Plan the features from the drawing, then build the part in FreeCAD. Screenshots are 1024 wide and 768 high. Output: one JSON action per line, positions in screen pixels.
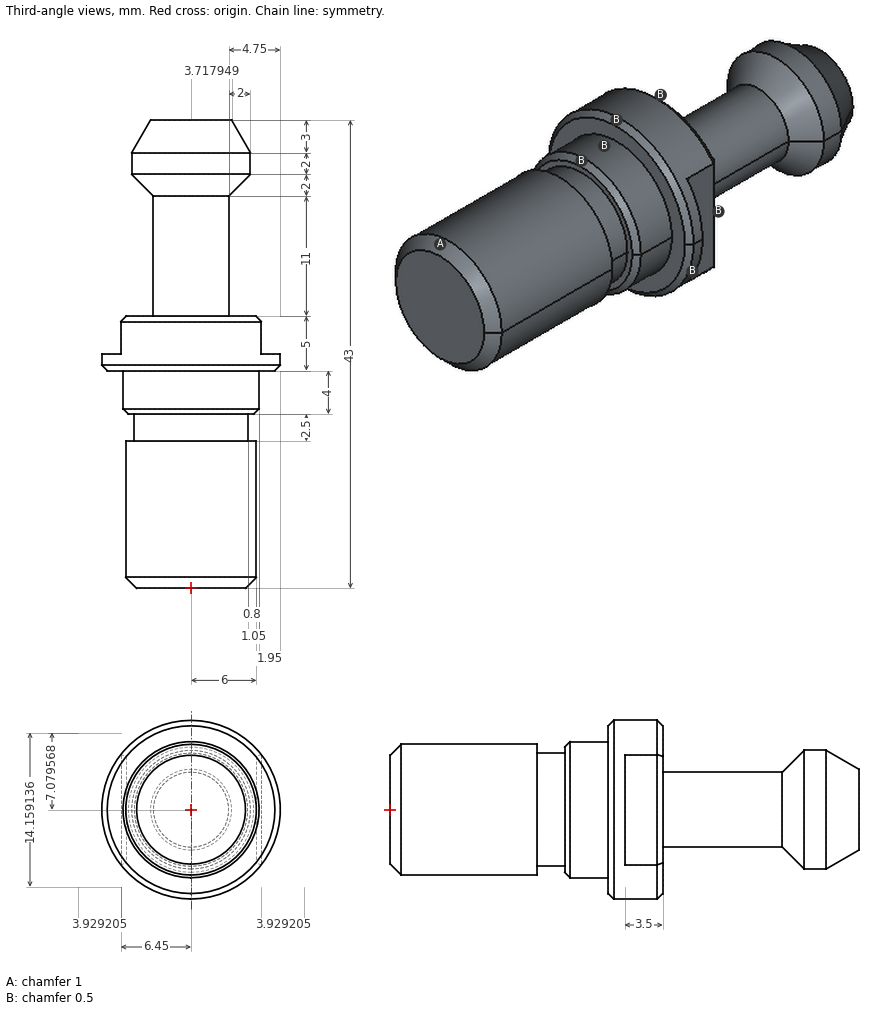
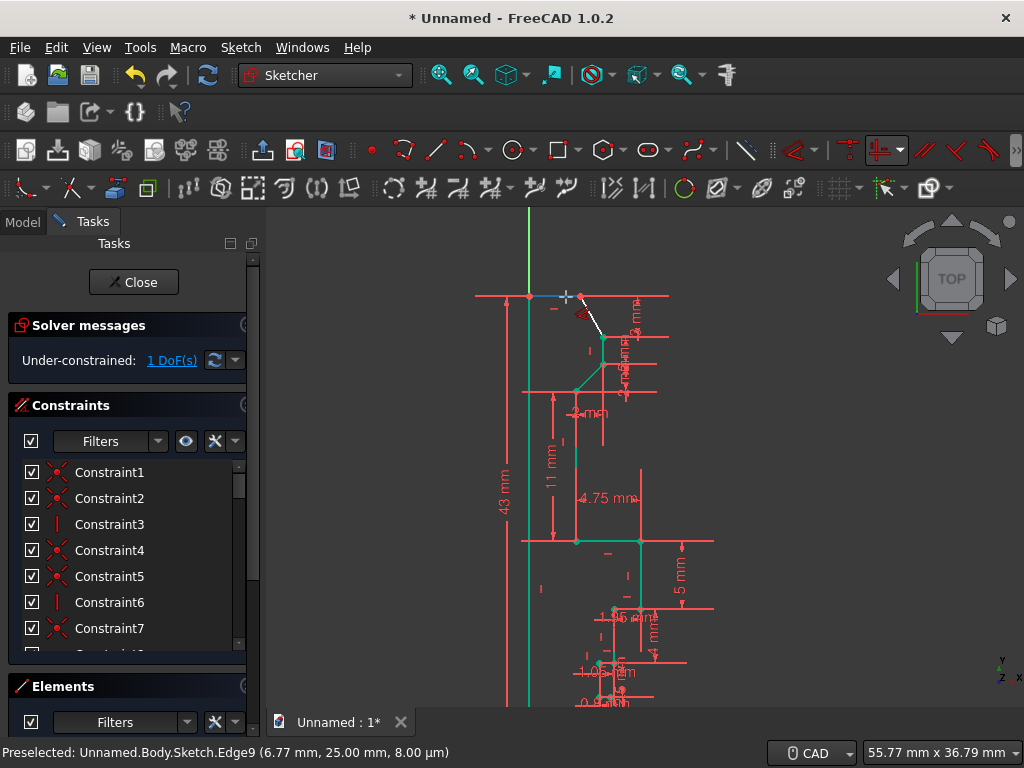
{"action": "left_click", "coordinate": [565, 296]}
{"action": "left_click", "coordinate": [555, 262]}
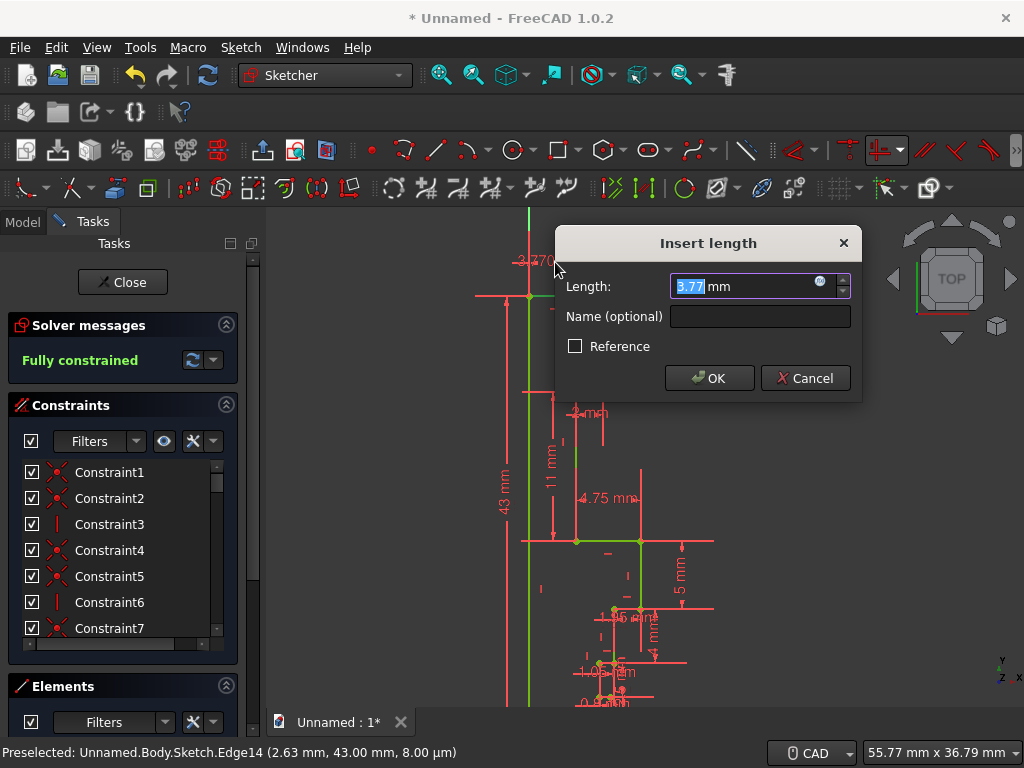
{"action": "type", "text": "3.717949"}
{"action": "key", "text": "Return"}
{"action": "key", "text": "Escape"}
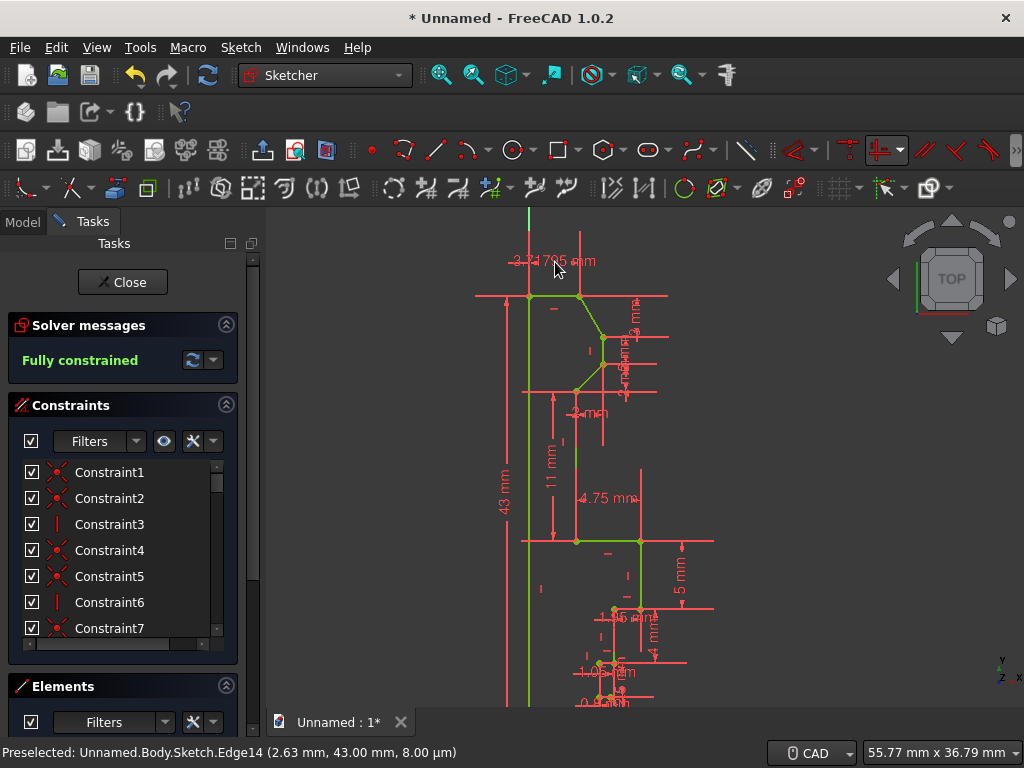
{"action": "left_click", "coordinate": [123, 282]}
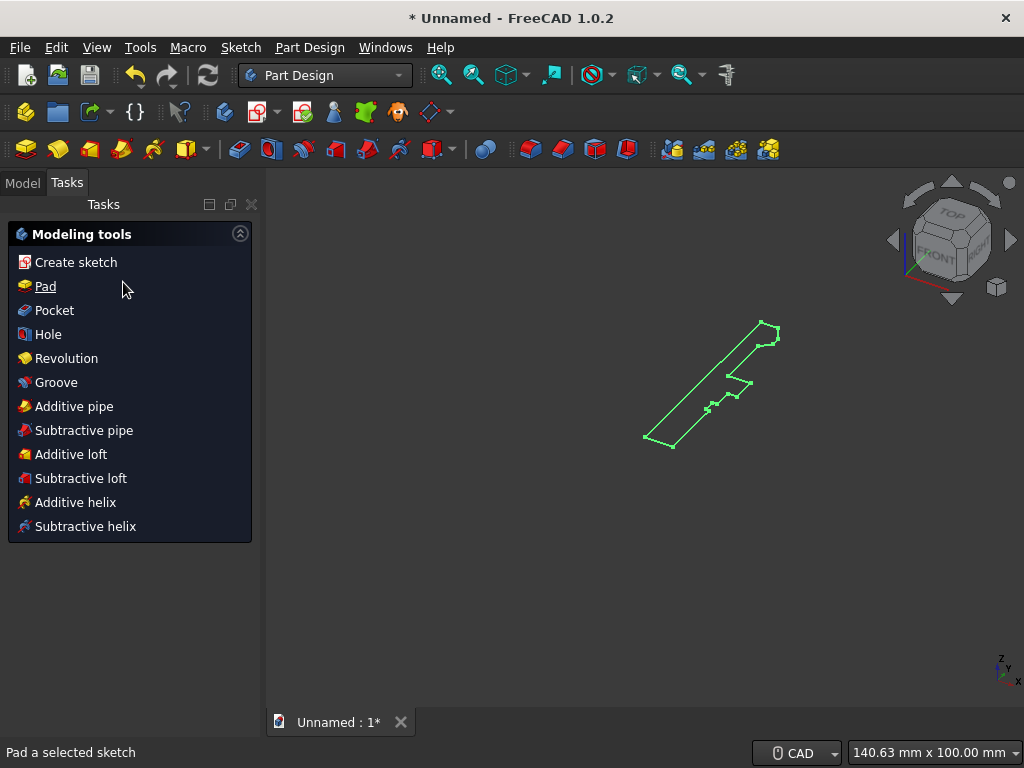
{"action": "left_click", "coordinate": [58, 150]}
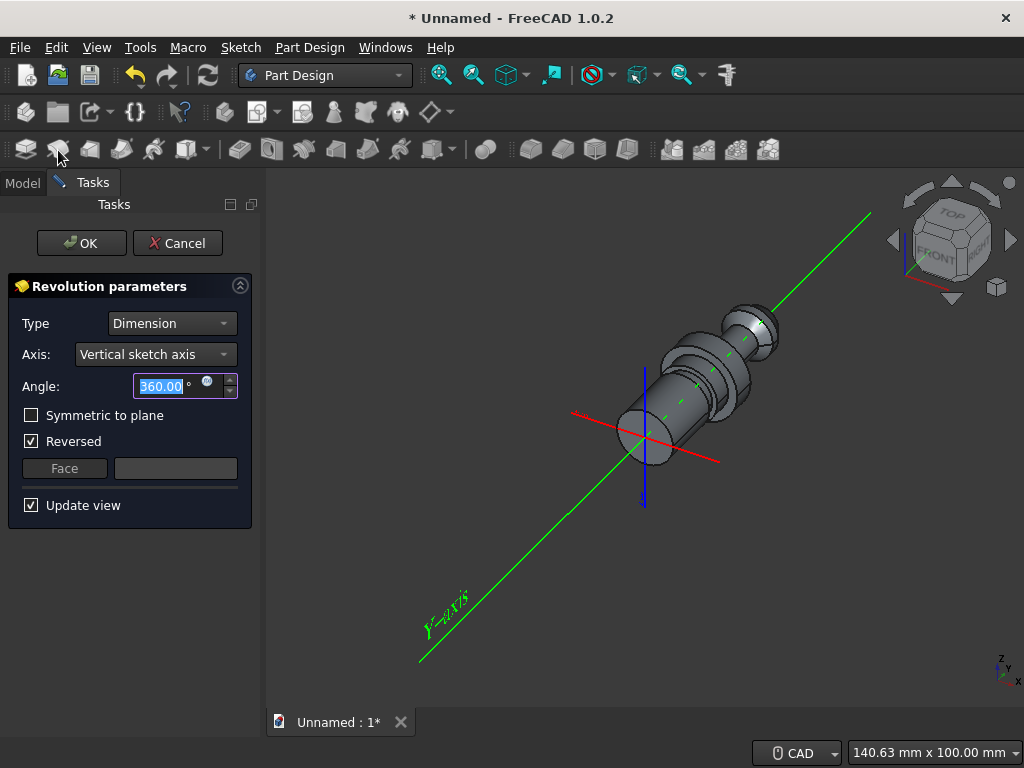
{"action": "left_click", "coordinate": [82, 243]}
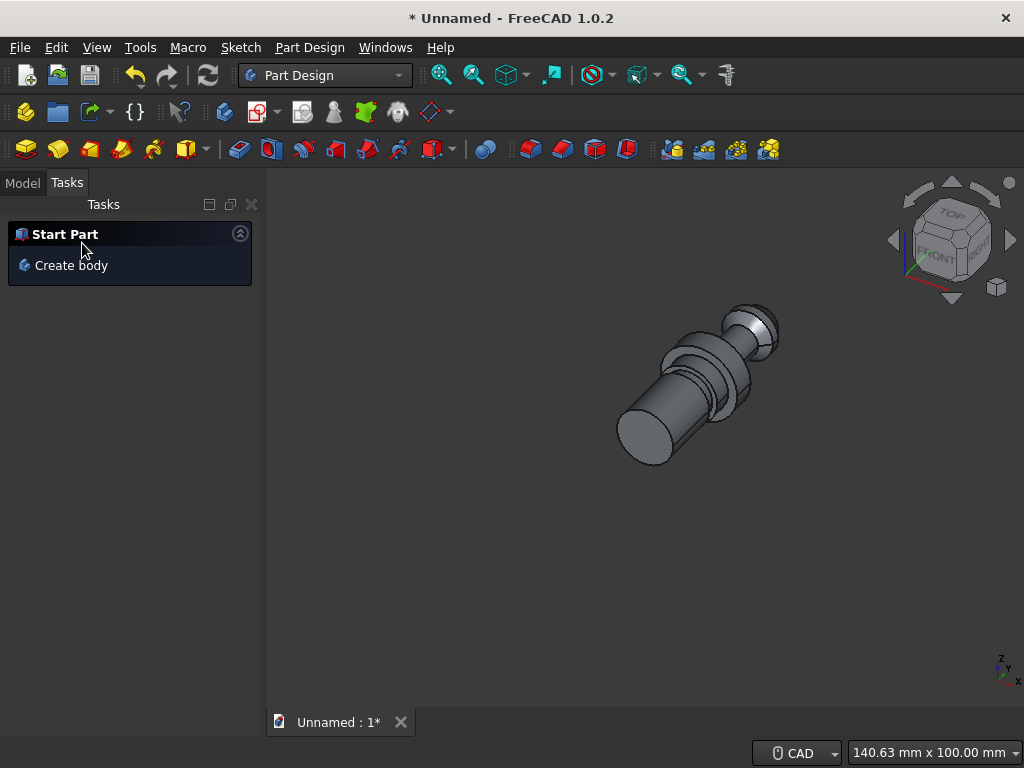
{"action": "left_click", "coordinate": [442, 76]}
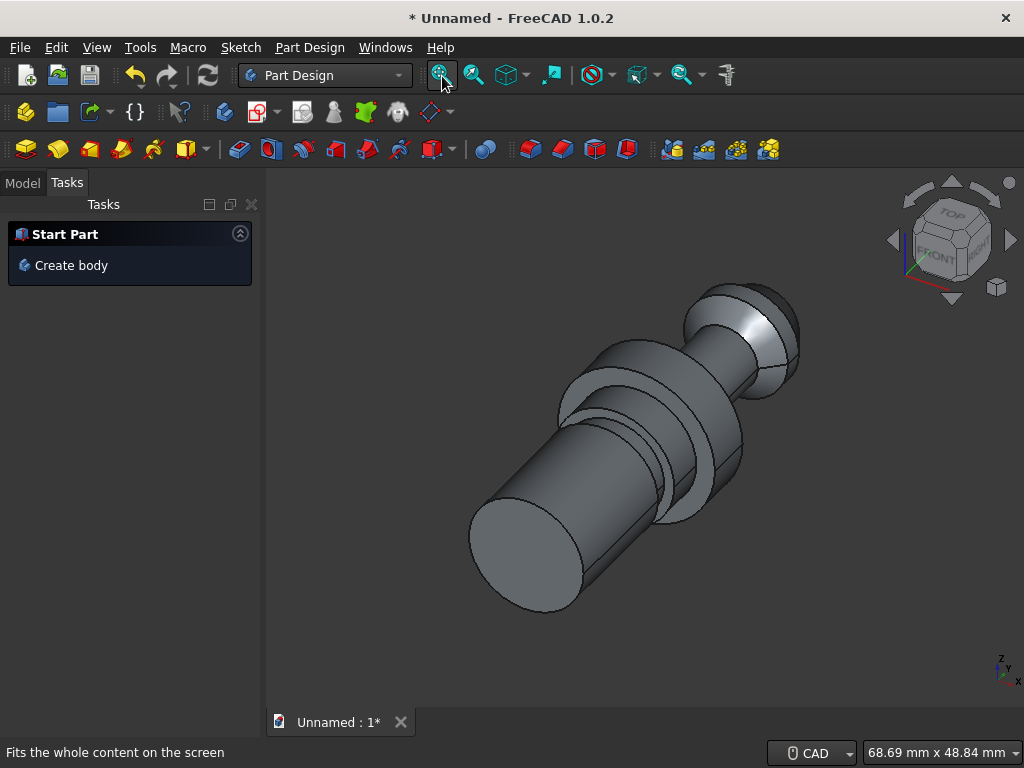
{"action": "left_click", "coordinate": [480, 507]}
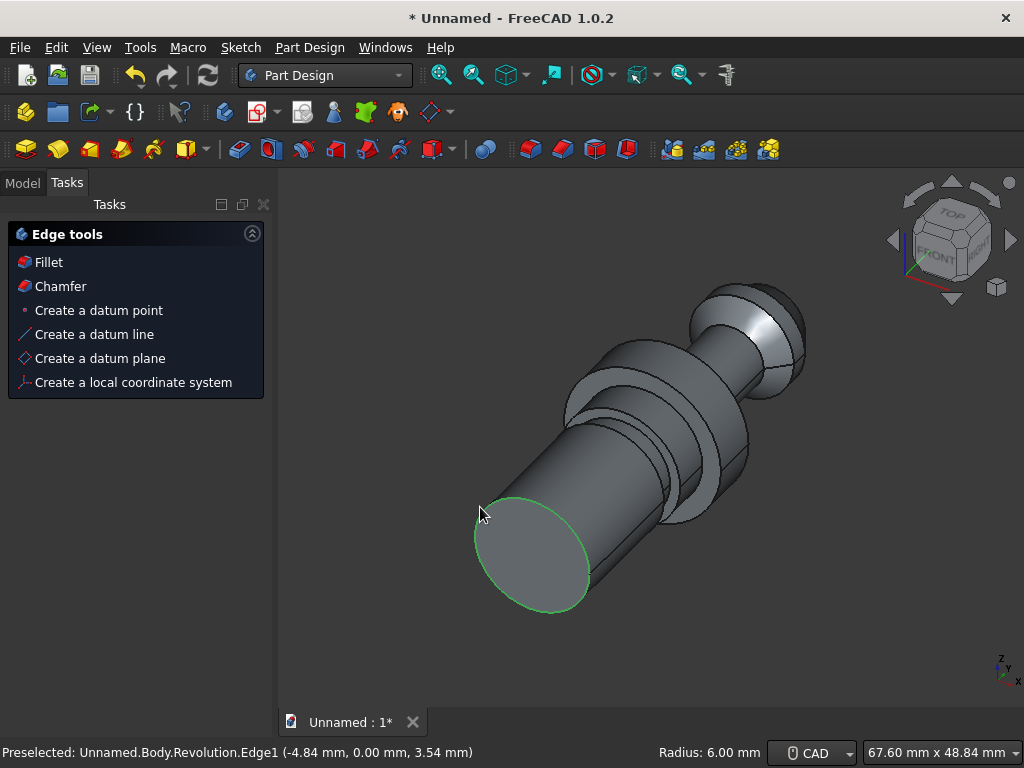
{"action": "left_click", "coordinate": [564, 150]}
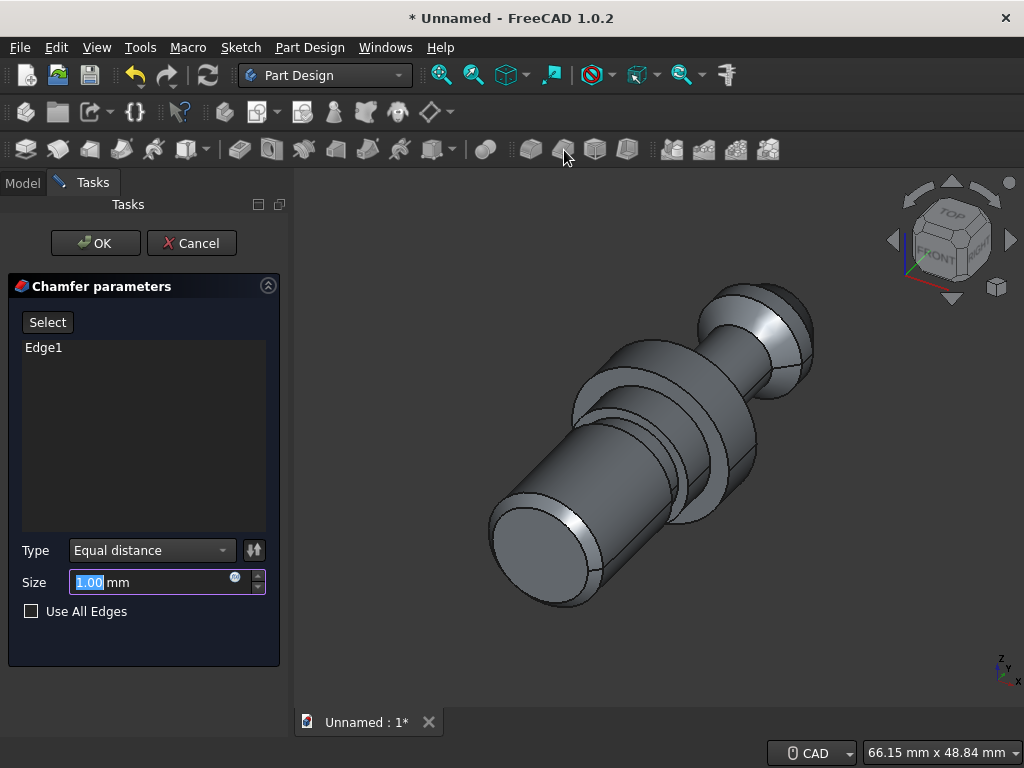
{"action": "type", "text": "1"}
{"action": "key", "text": "Tab"}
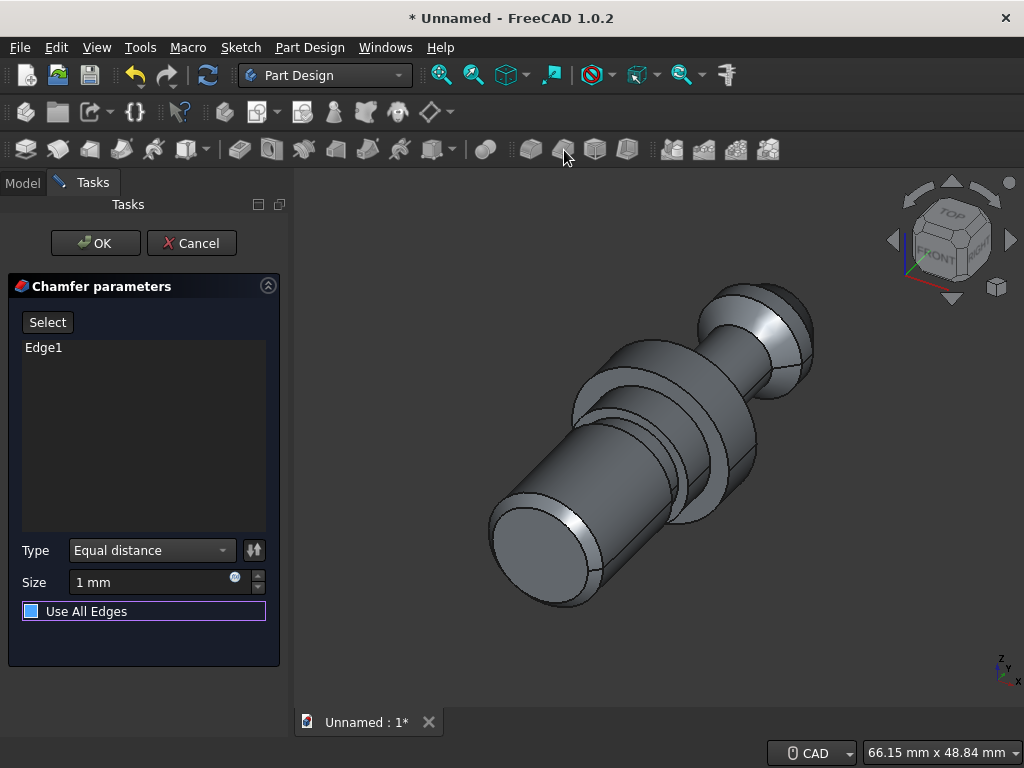
{"action": "left_click", "coordinate": [96, 243]}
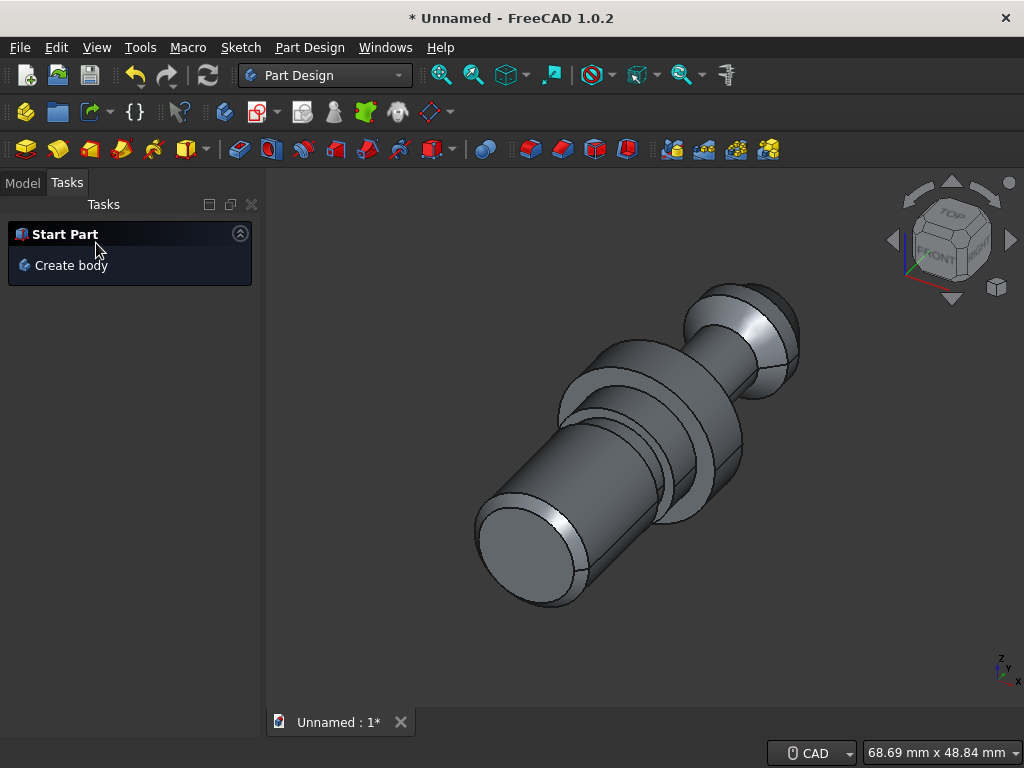
{"action": "left_click", "coordinate": [23, 182]}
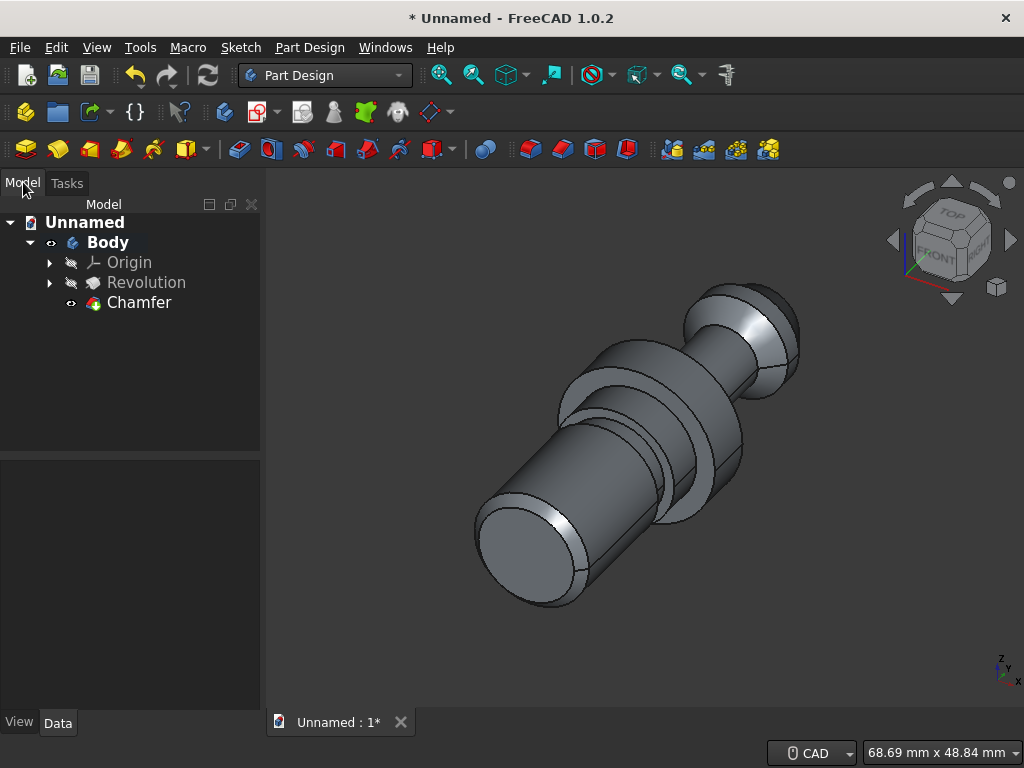
{"action": "left_click", "coordinate": [50, 263]}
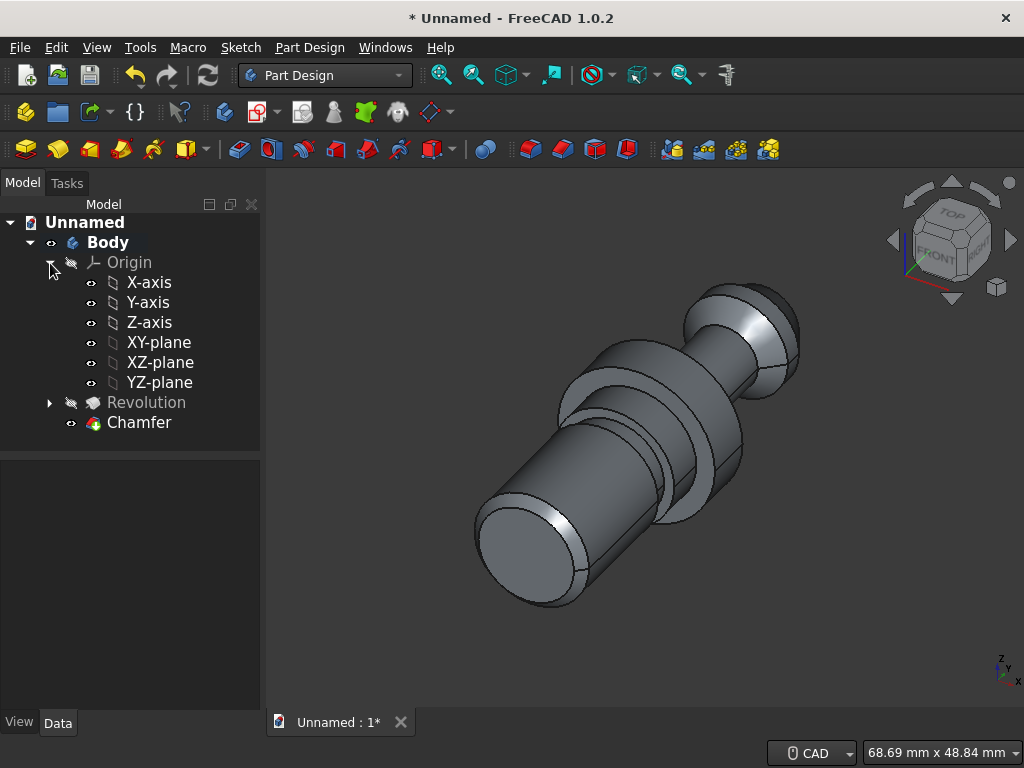
{"action": "left_click", "coordinate": [136, 363]}